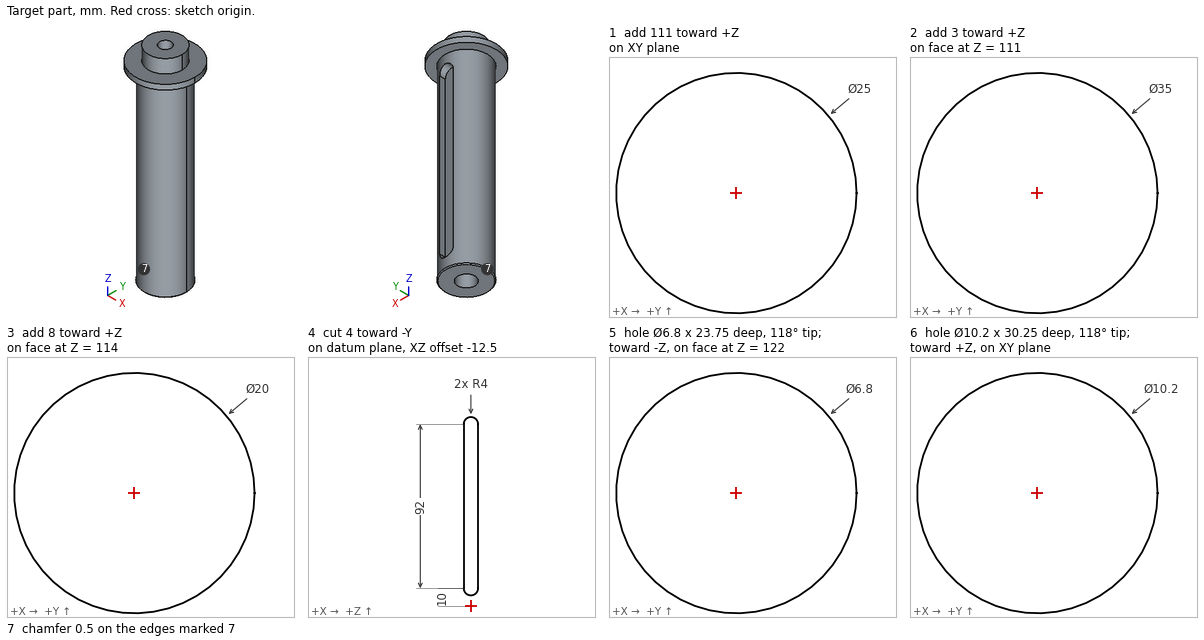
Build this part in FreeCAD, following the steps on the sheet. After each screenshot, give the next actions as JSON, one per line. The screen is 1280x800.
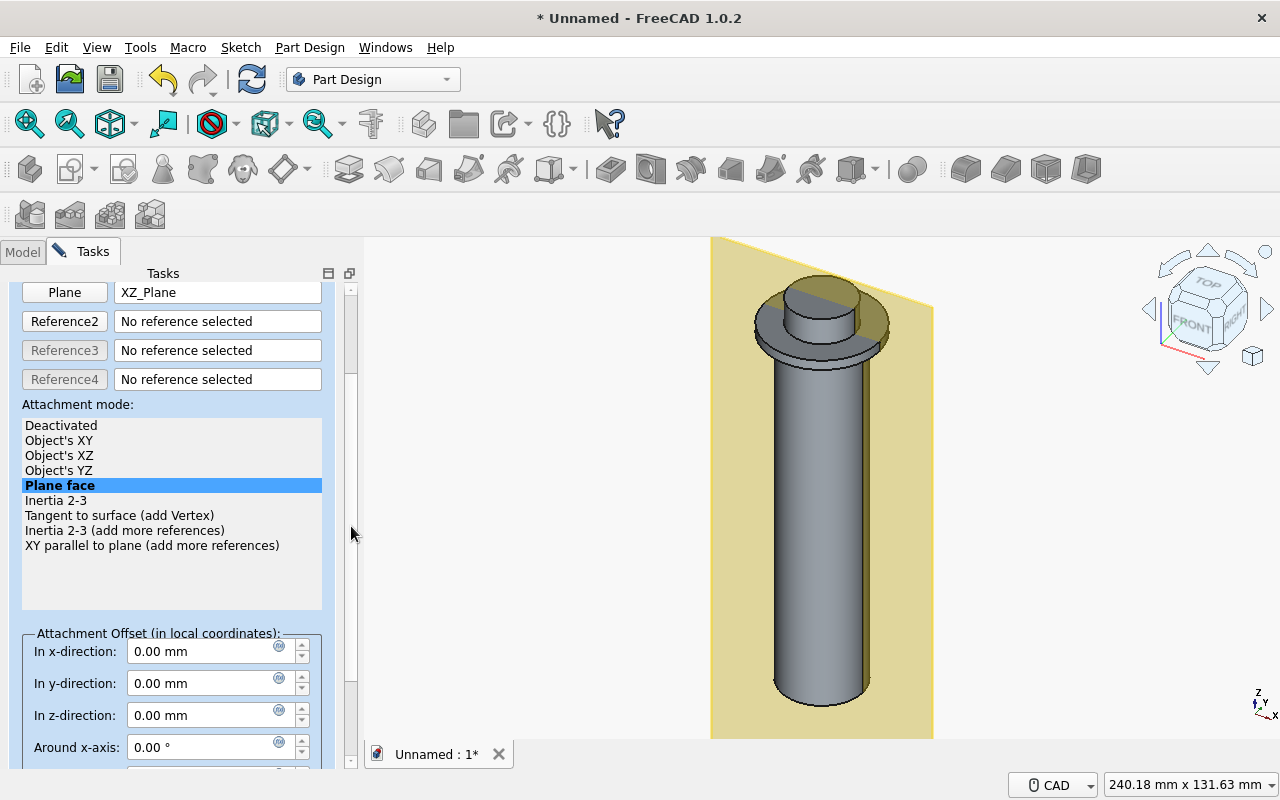
{"action": "triple_click", "coordinate": [210, 655]}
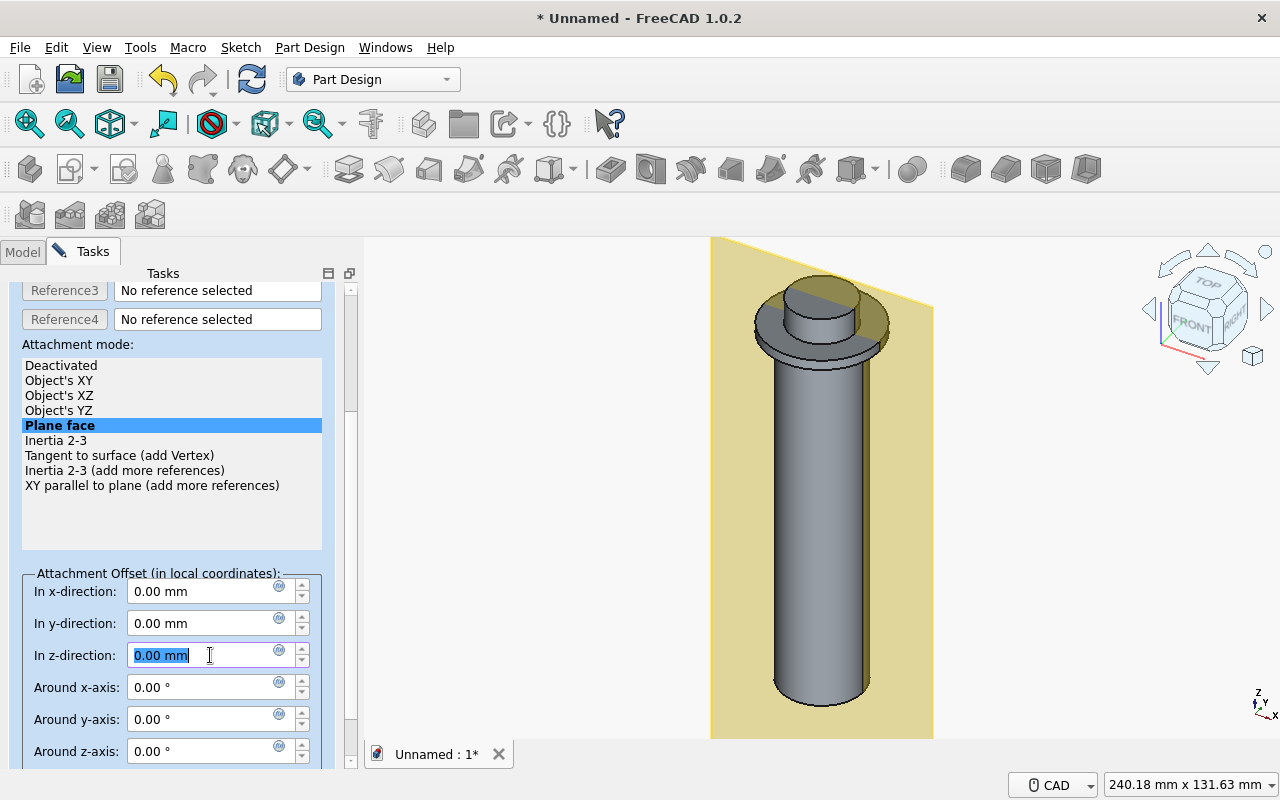
{"action": "type", "text": "-12.5"}
{"action": "key", "text": "Tab"}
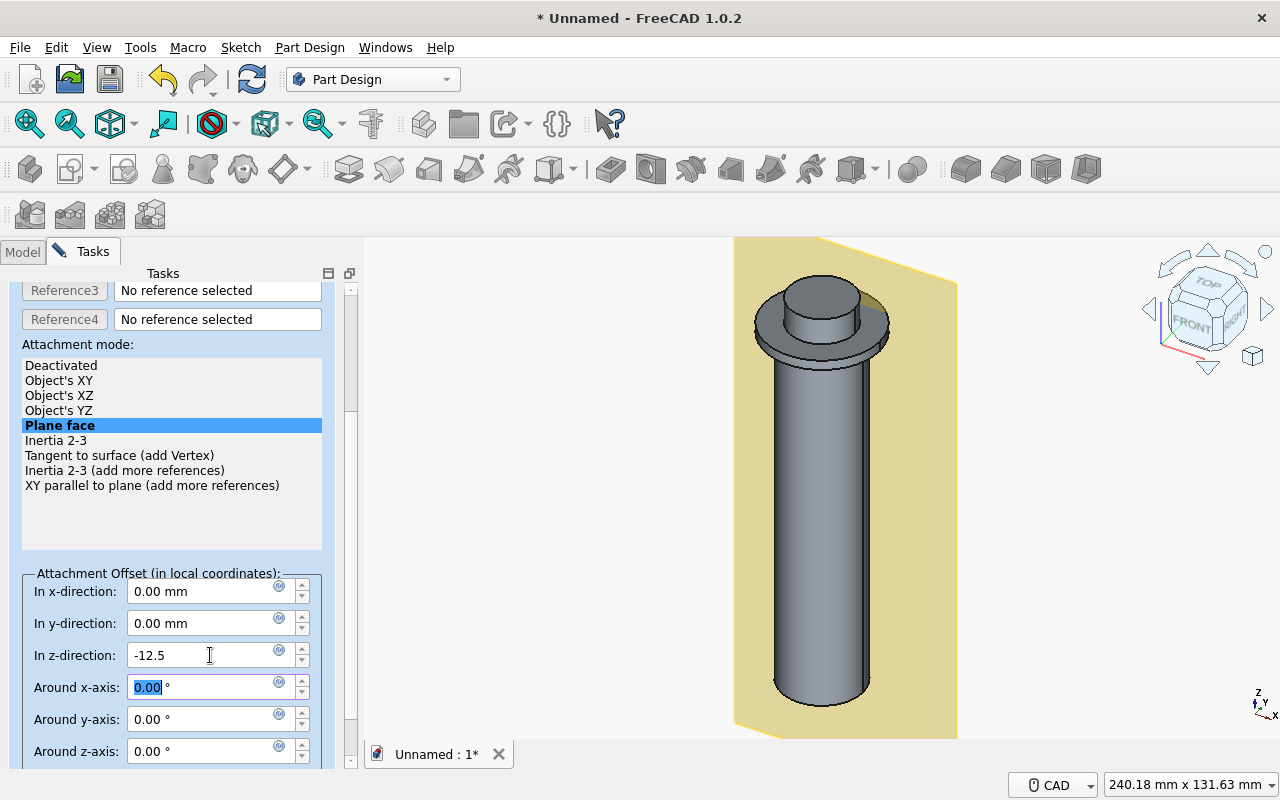
{"action": "scroll", "coordinate": [351, 526], "scroll_direction": "up", "scroll_amount": 4}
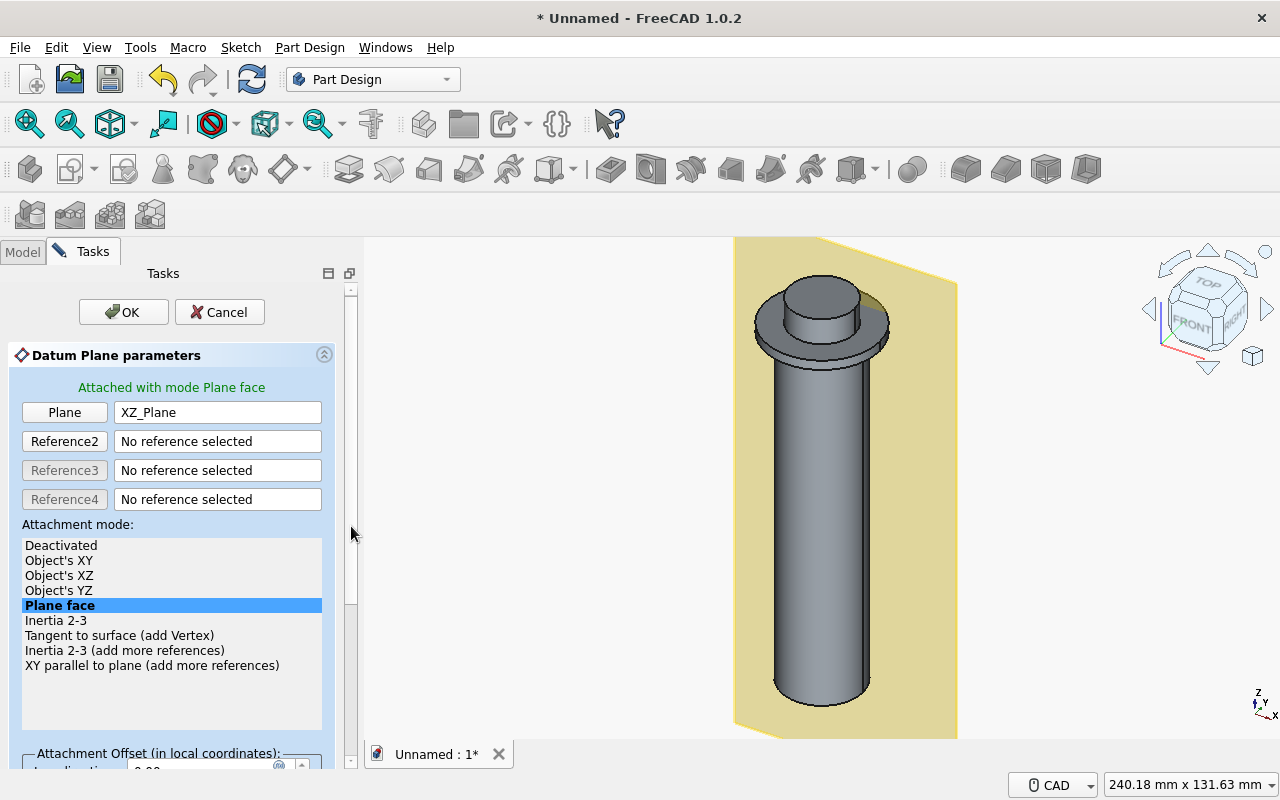
{"action": "left_click", "coordinate": [124, 312]}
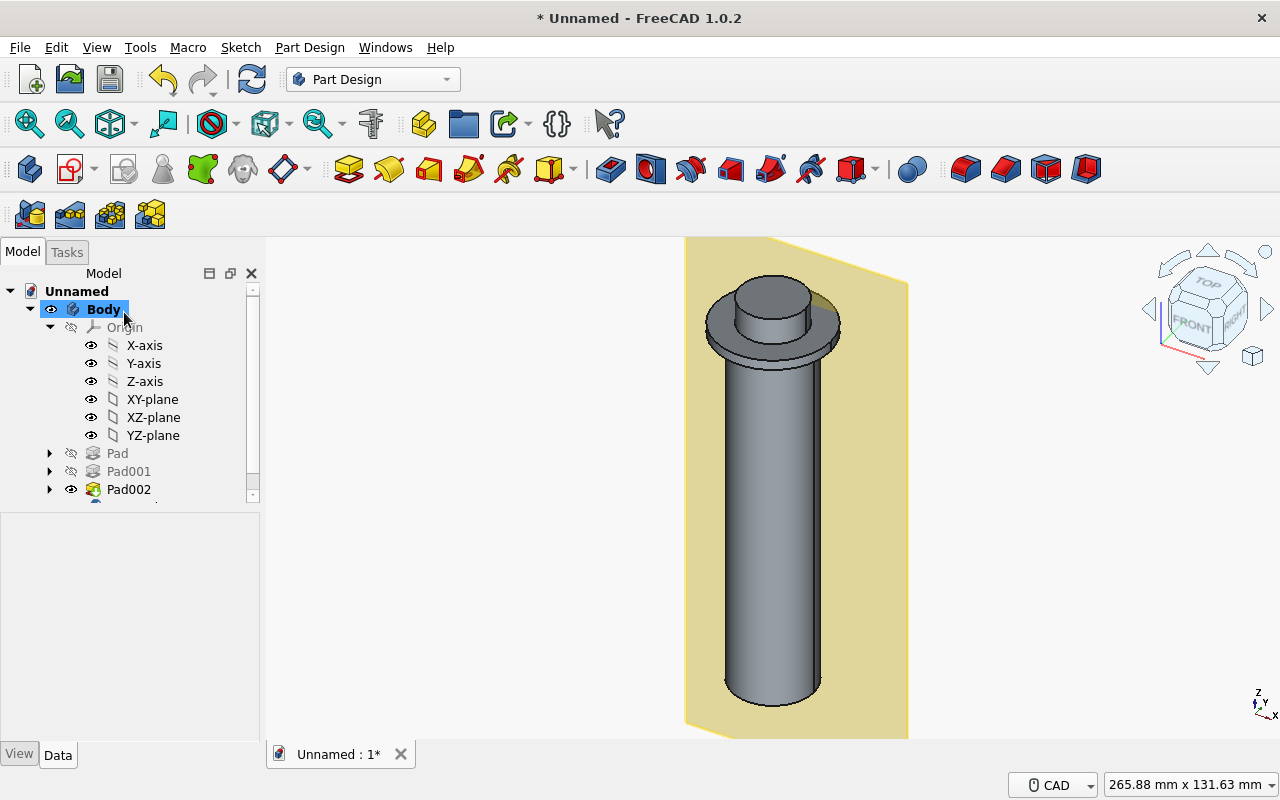
{"action": "scroll", "coordinate": [100, 395], "scroll_direction": "down", "scroll_amount": 3}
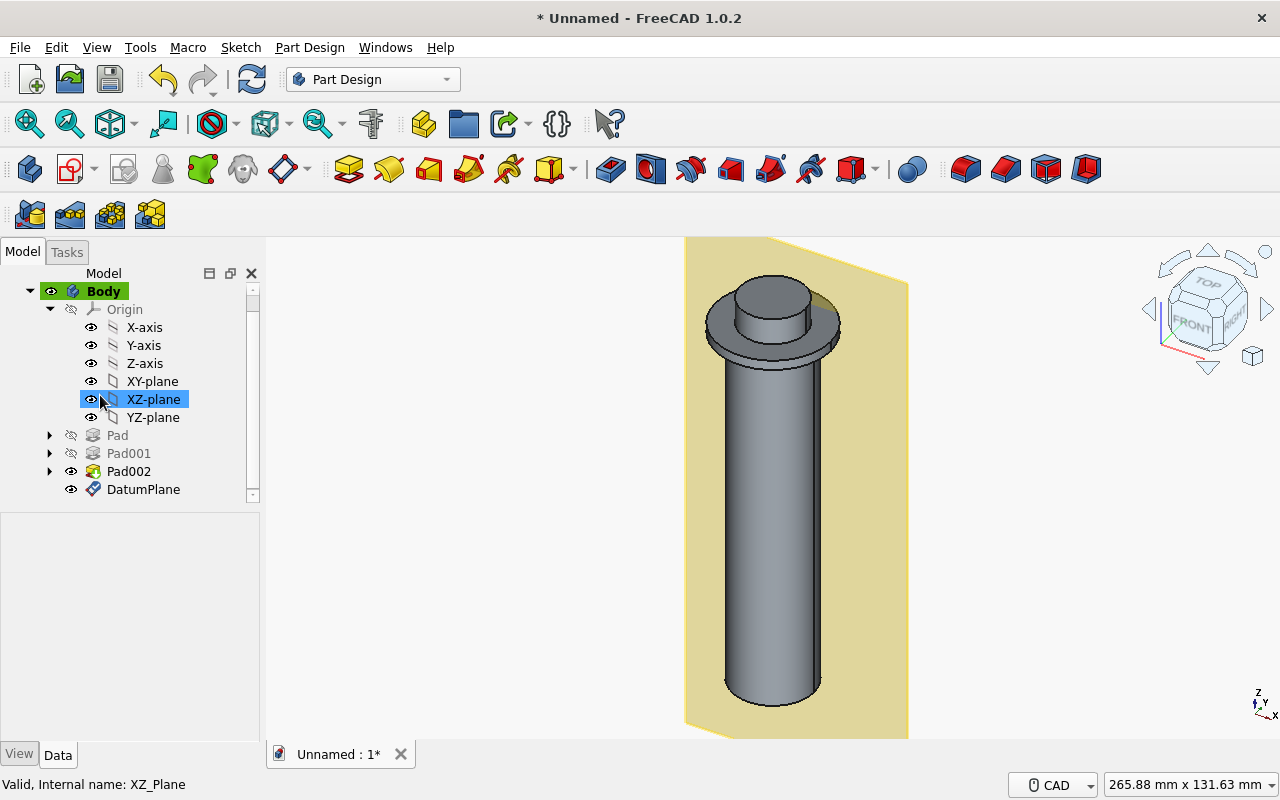
{"action": "left_click", "coordinate": [116, 489]}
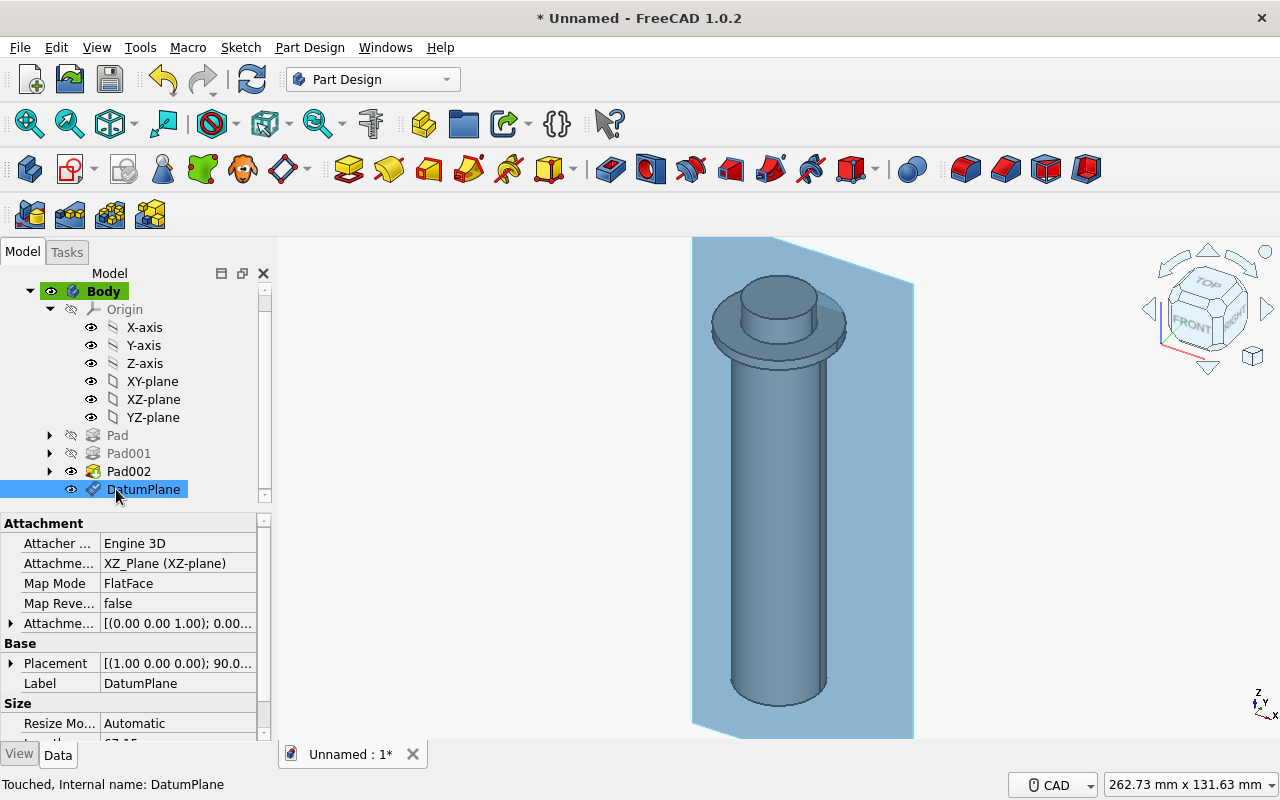
{"action": "left_click", "coordinate": [70, 170]}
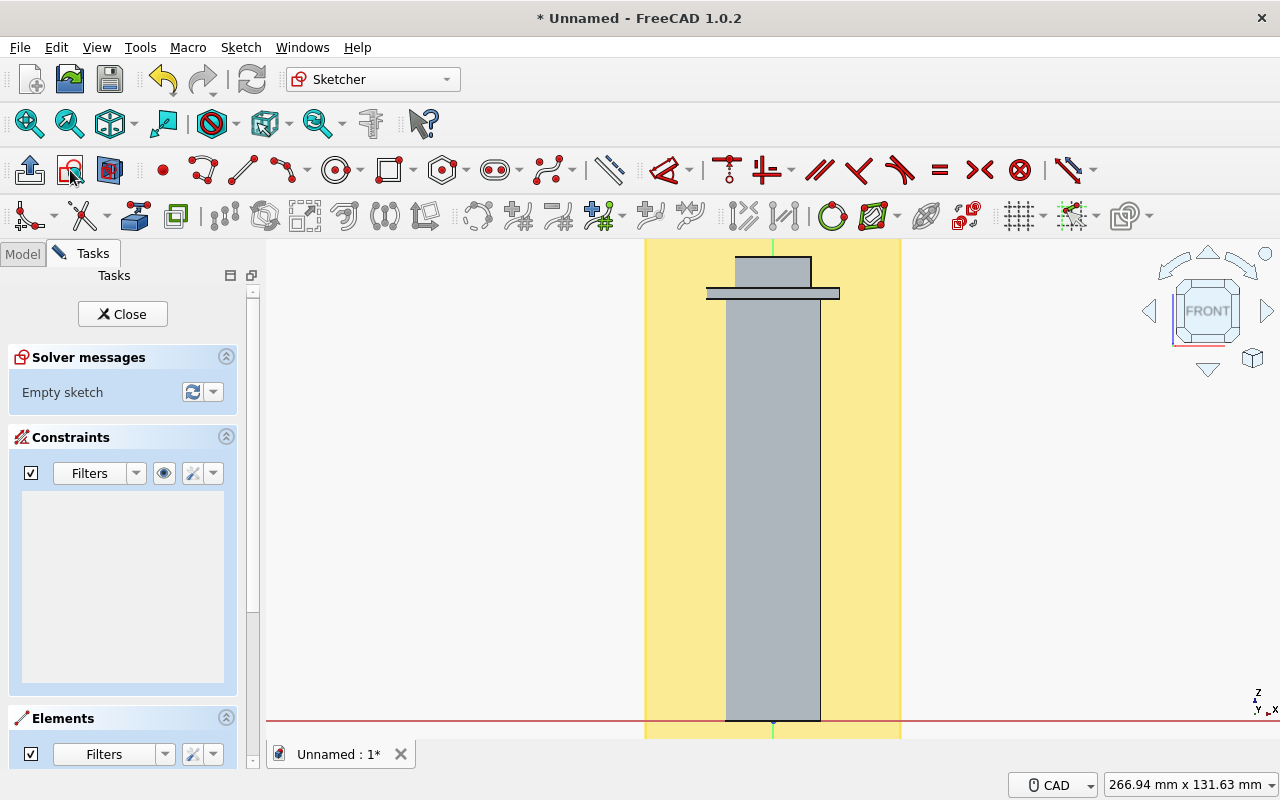
{"action": "left_click", "coordinate": [110, 170]}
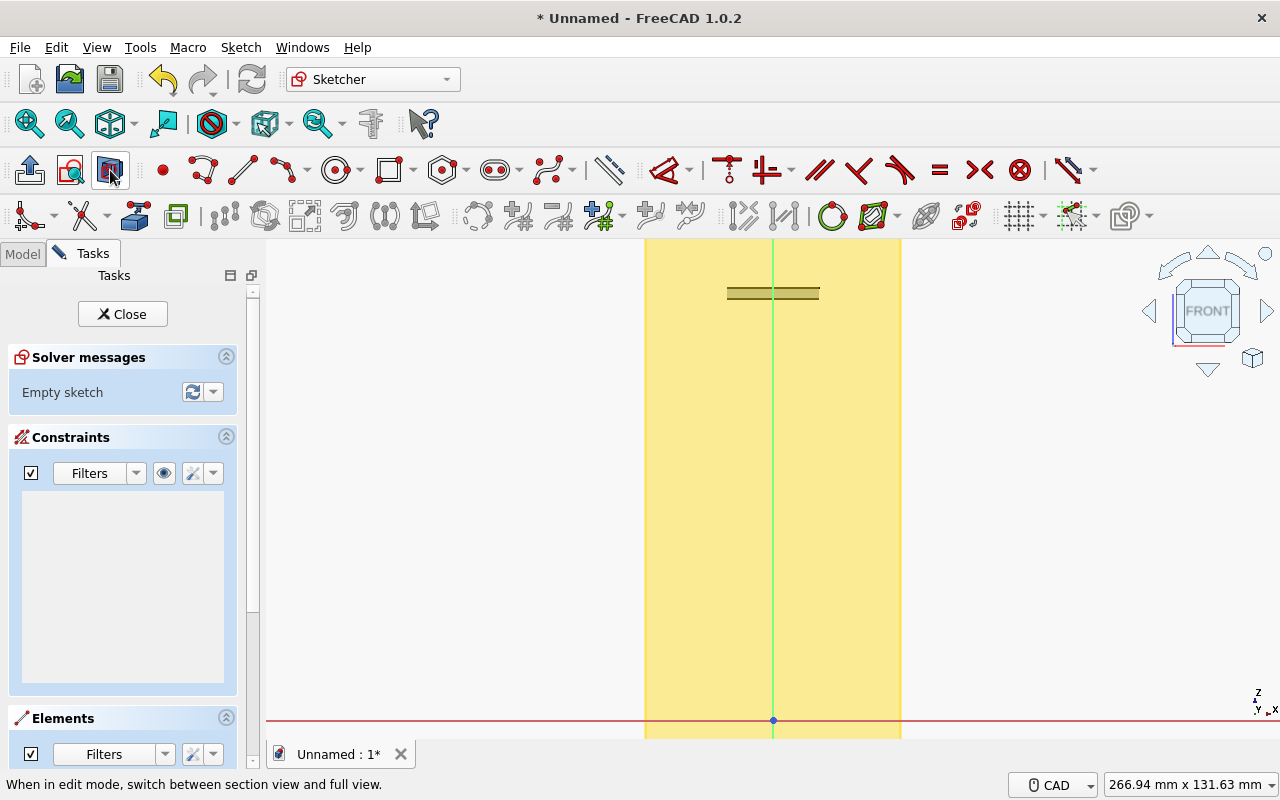
{"action": "scroll", "coordinate": [395, 352], "scroll_direction": "down", "scroll_amount": 1}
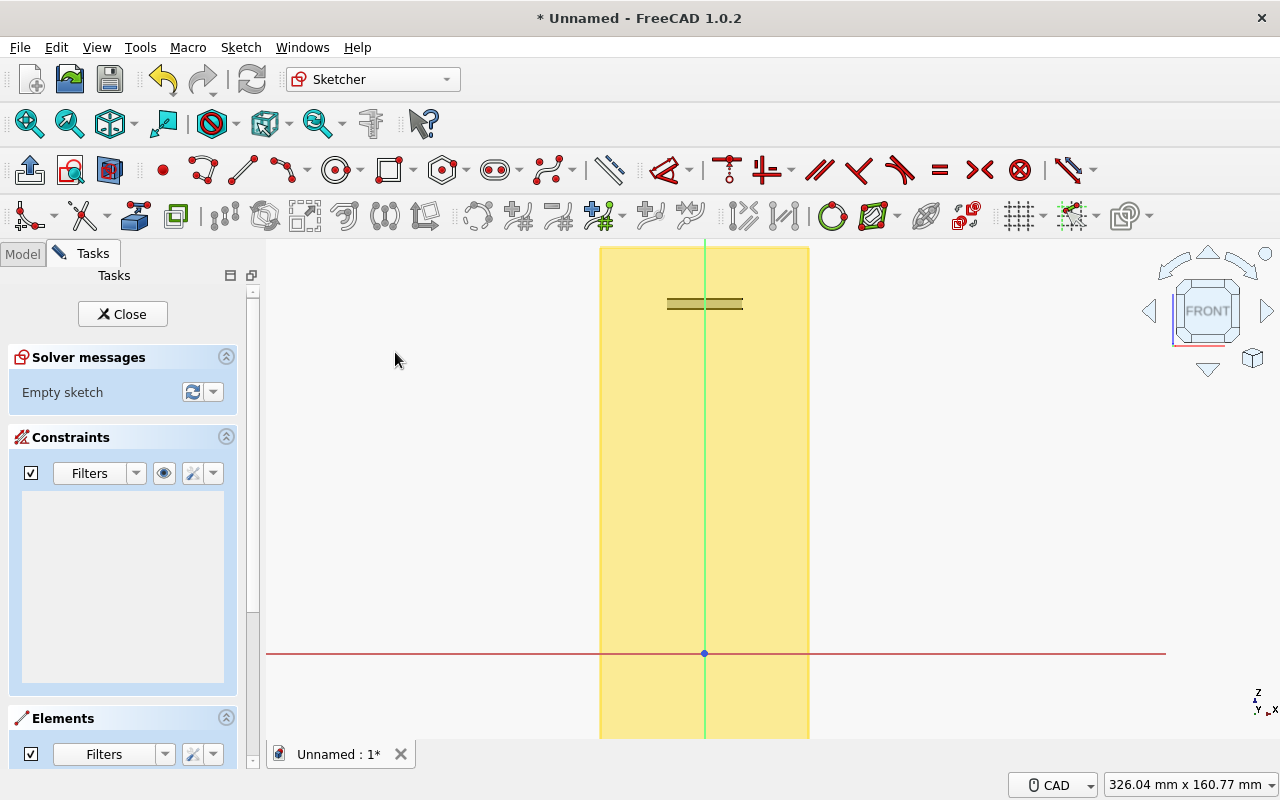
{"action": "left_click", "coordinate": [496, 170]}